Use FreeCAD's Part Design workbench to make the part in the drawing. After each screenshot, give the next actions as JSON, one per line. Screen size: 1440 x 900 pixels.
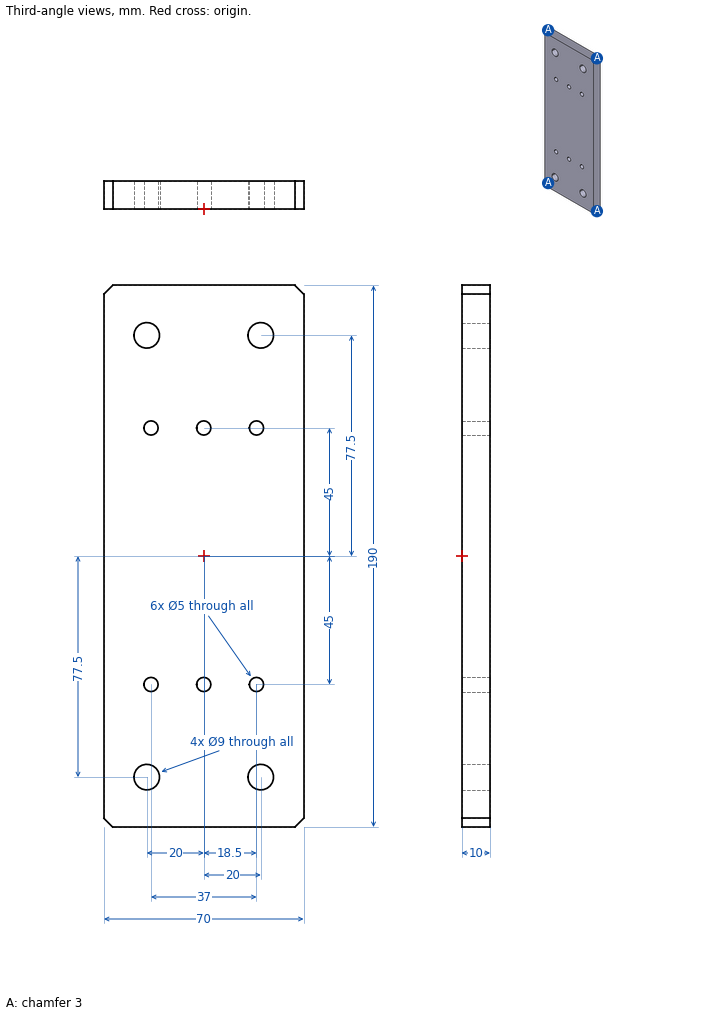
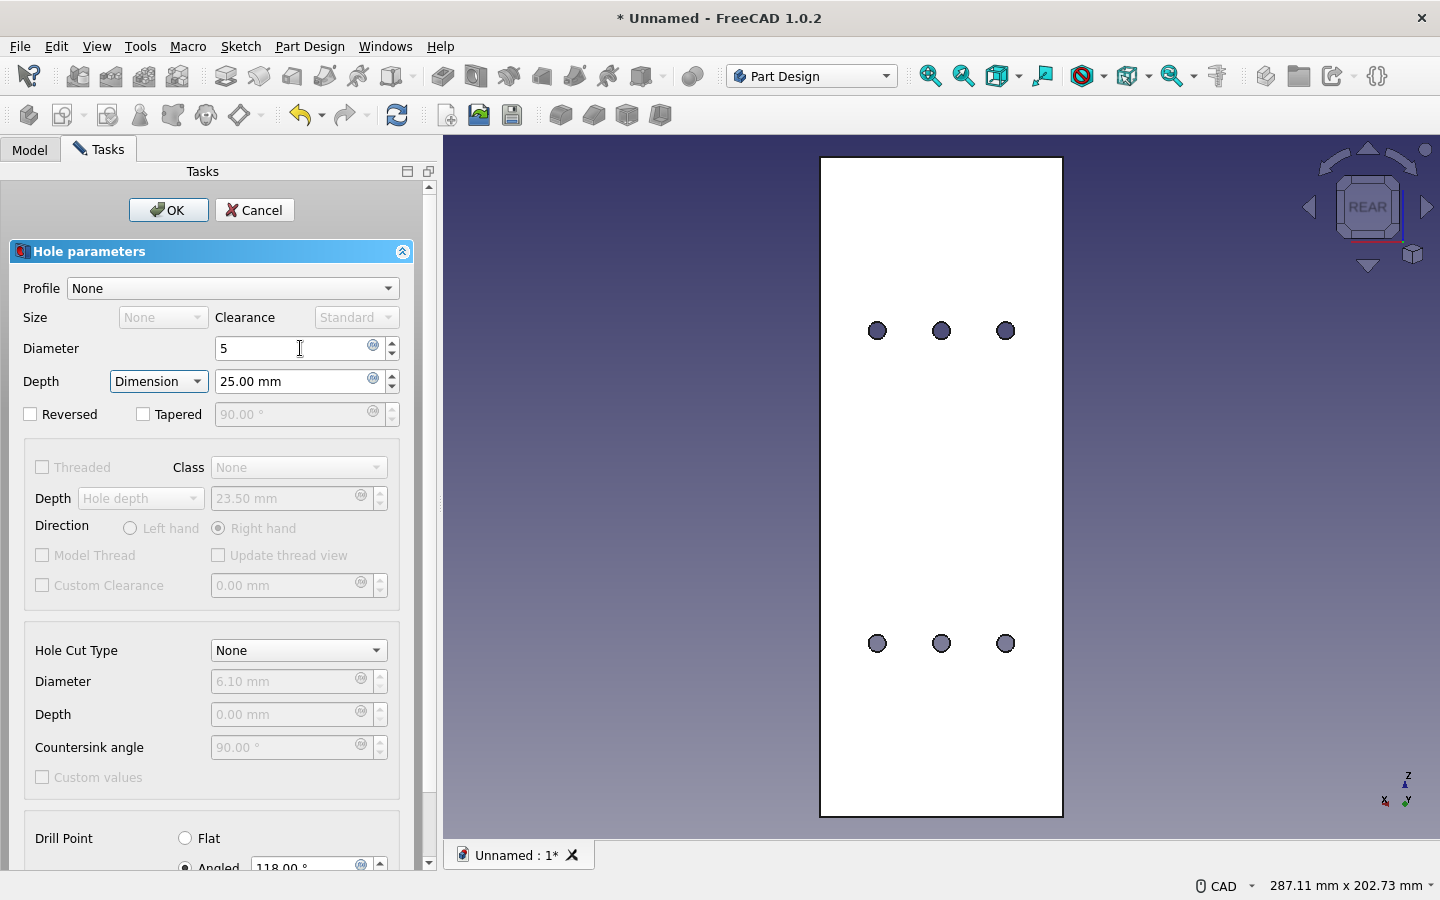
{"action": "left_click", "coordinate": [160, 382]}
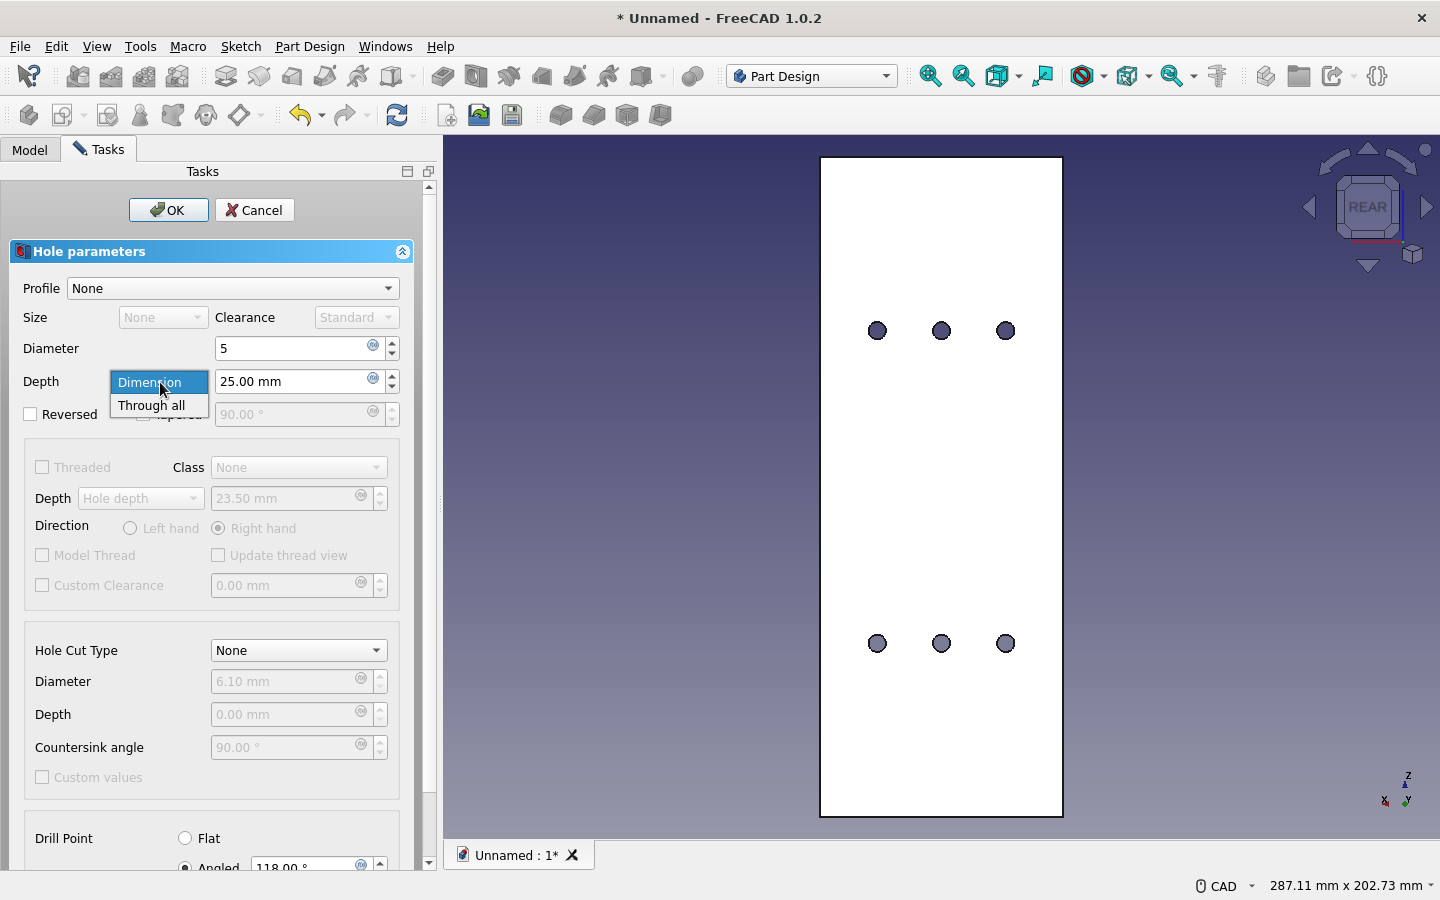
{"action": "left_click", "coordinate": [158, 406]}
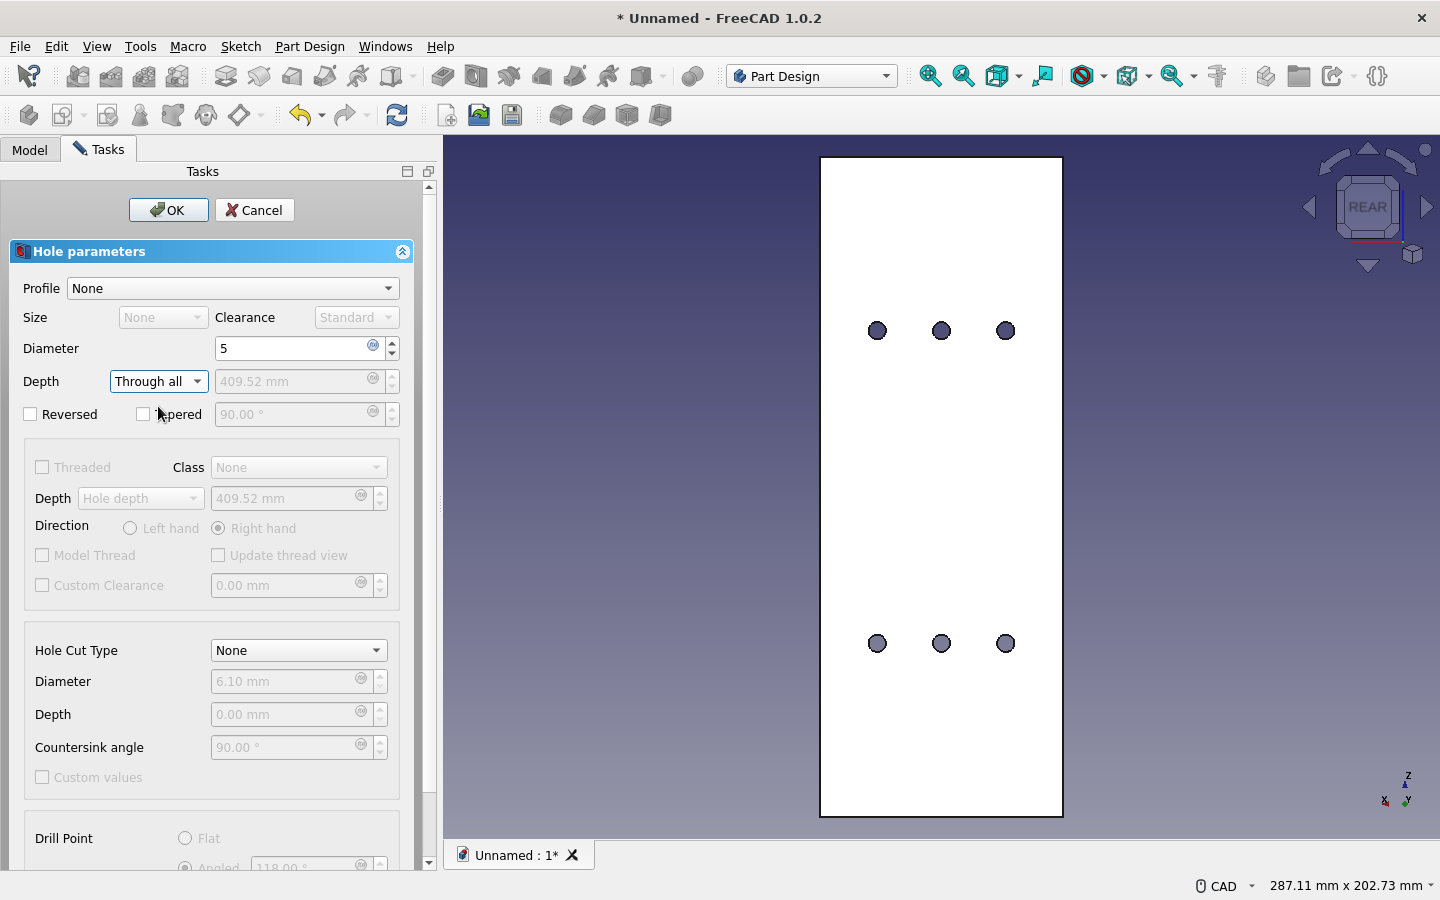
{"action": "left_click", "coordinate": [169, 210]}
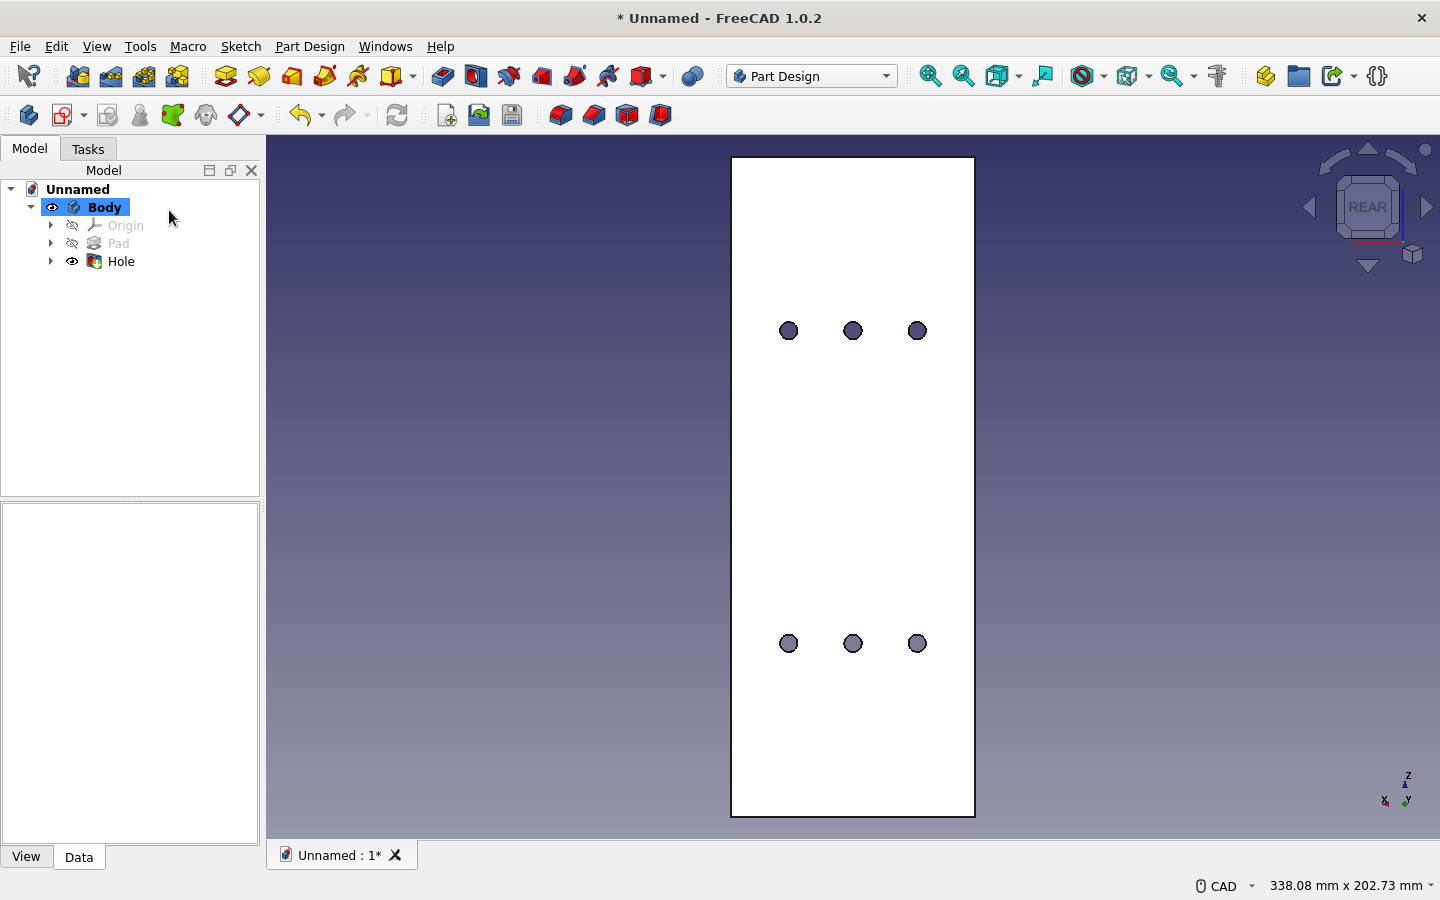
{"action": "left_click", "coordinate": [853, 486]}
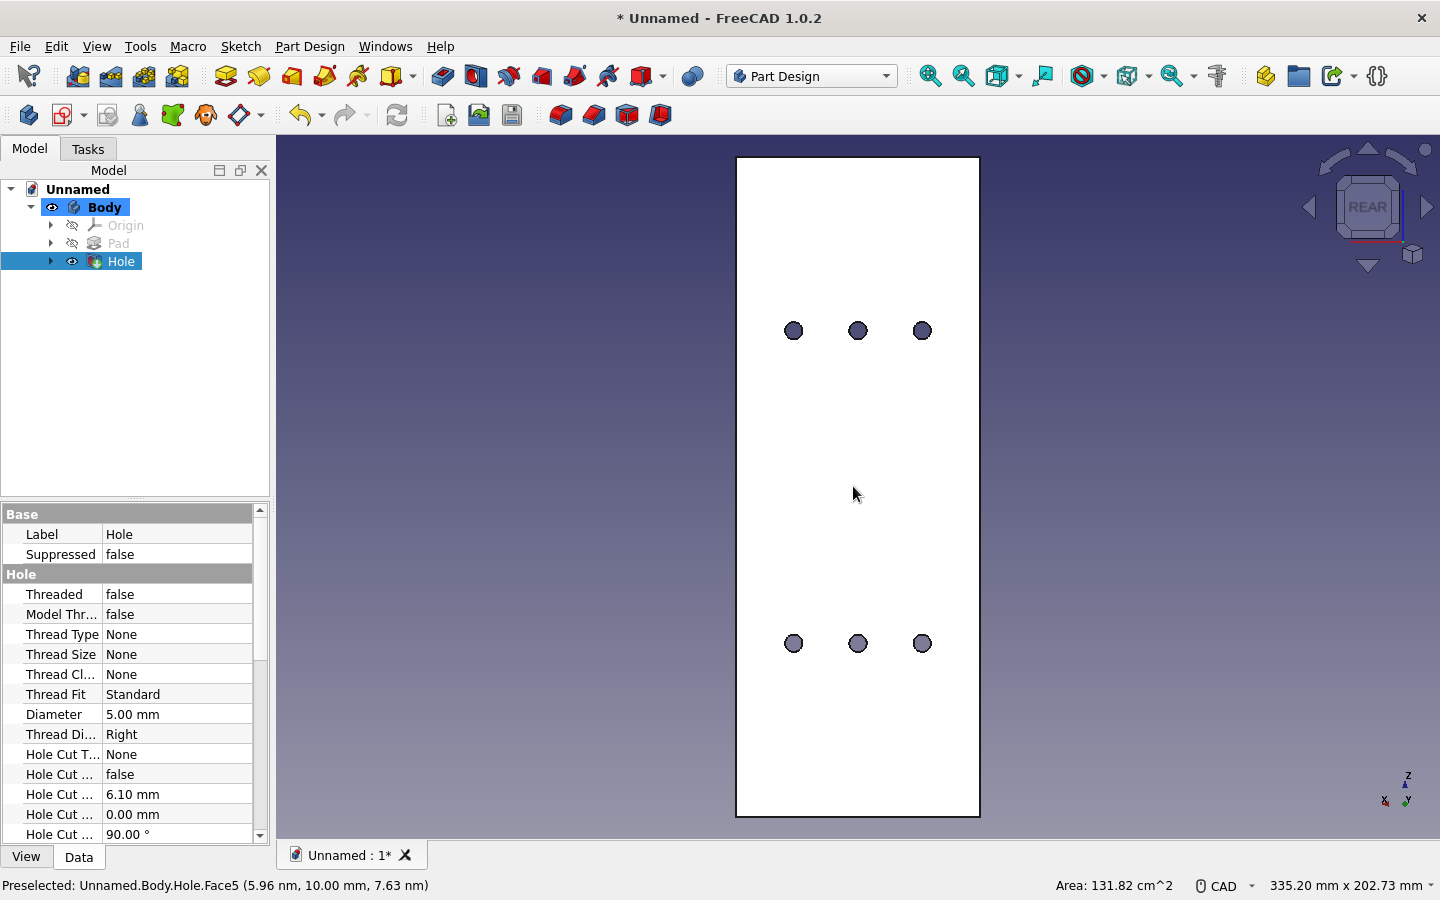
{"action": "left_click", "coordinate": [62, 116]}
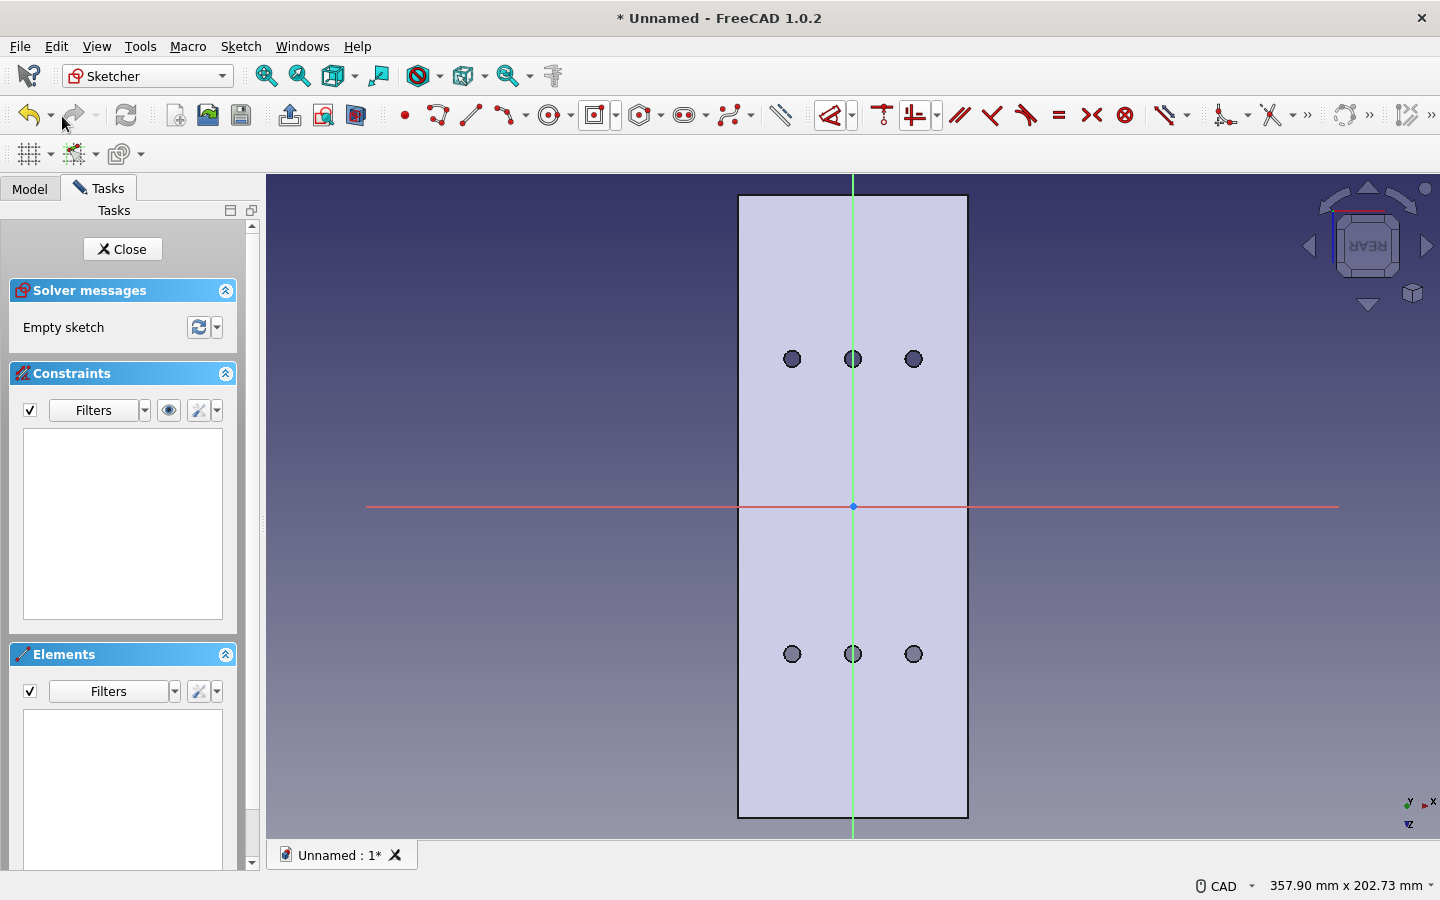
{"action": "left_click", "coordinate": [548, 116]}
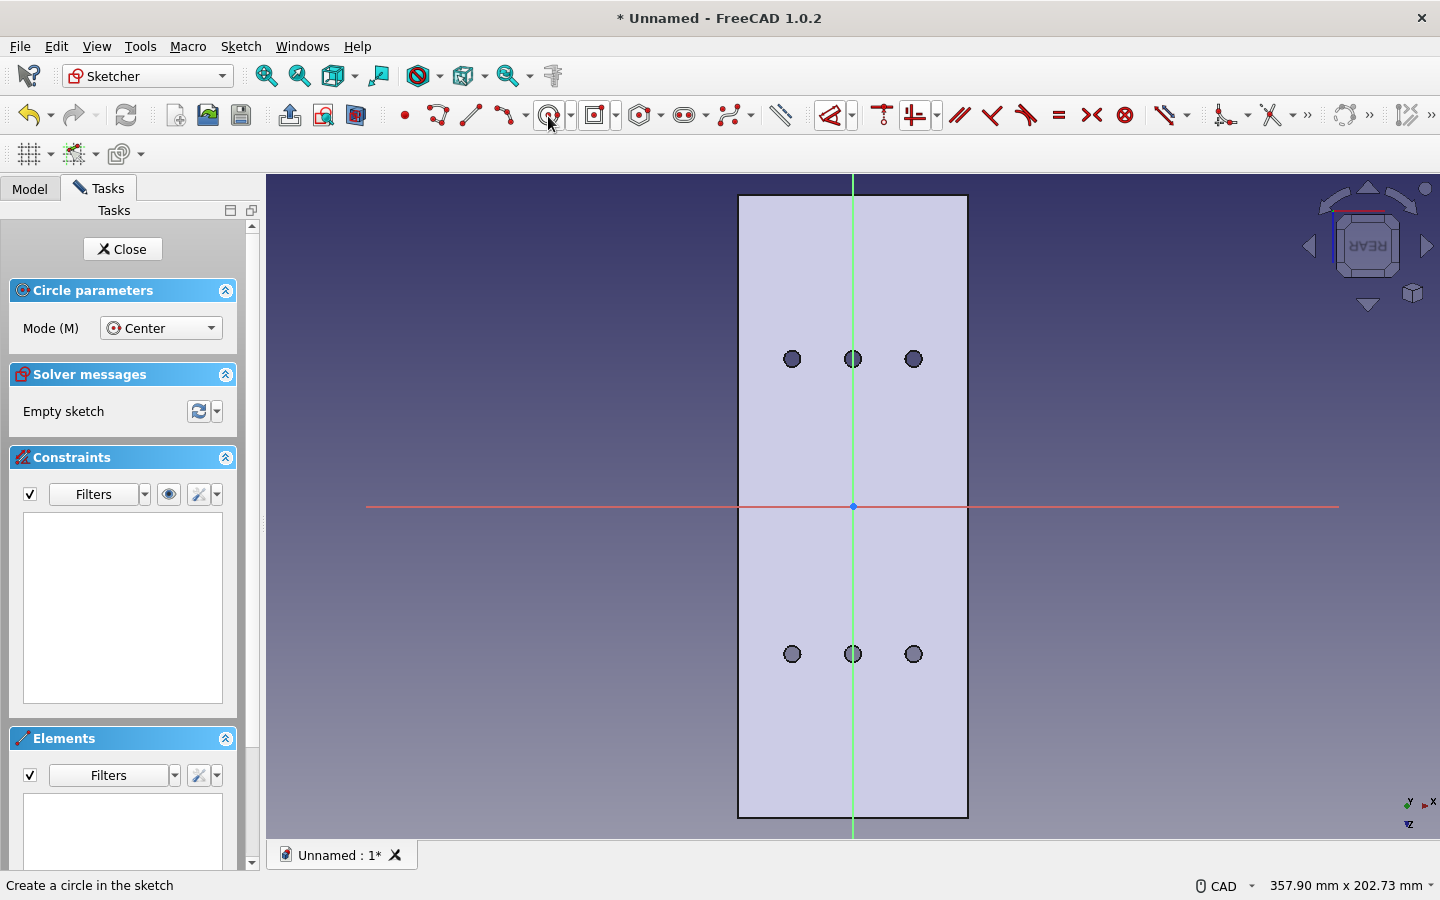
{"action": "scroll", "coordinate": [787, 252], "scroll_direction": "up", "scroll_amount": 3}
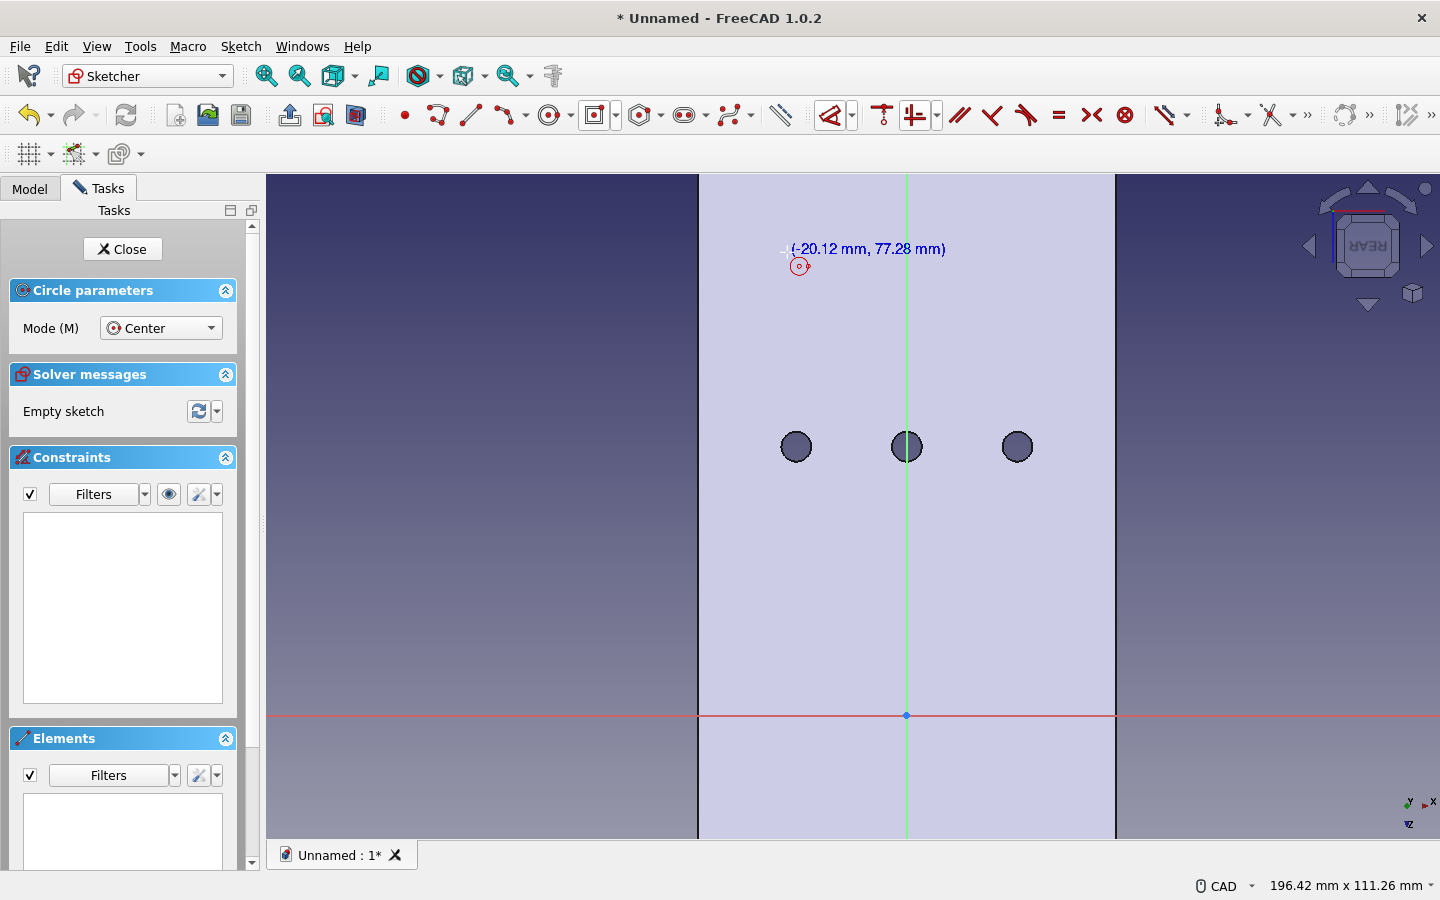
{"action": "left_click", "coordinate": [787, 252]}
{"action": "left_click", "coordinate": [806, 233]}